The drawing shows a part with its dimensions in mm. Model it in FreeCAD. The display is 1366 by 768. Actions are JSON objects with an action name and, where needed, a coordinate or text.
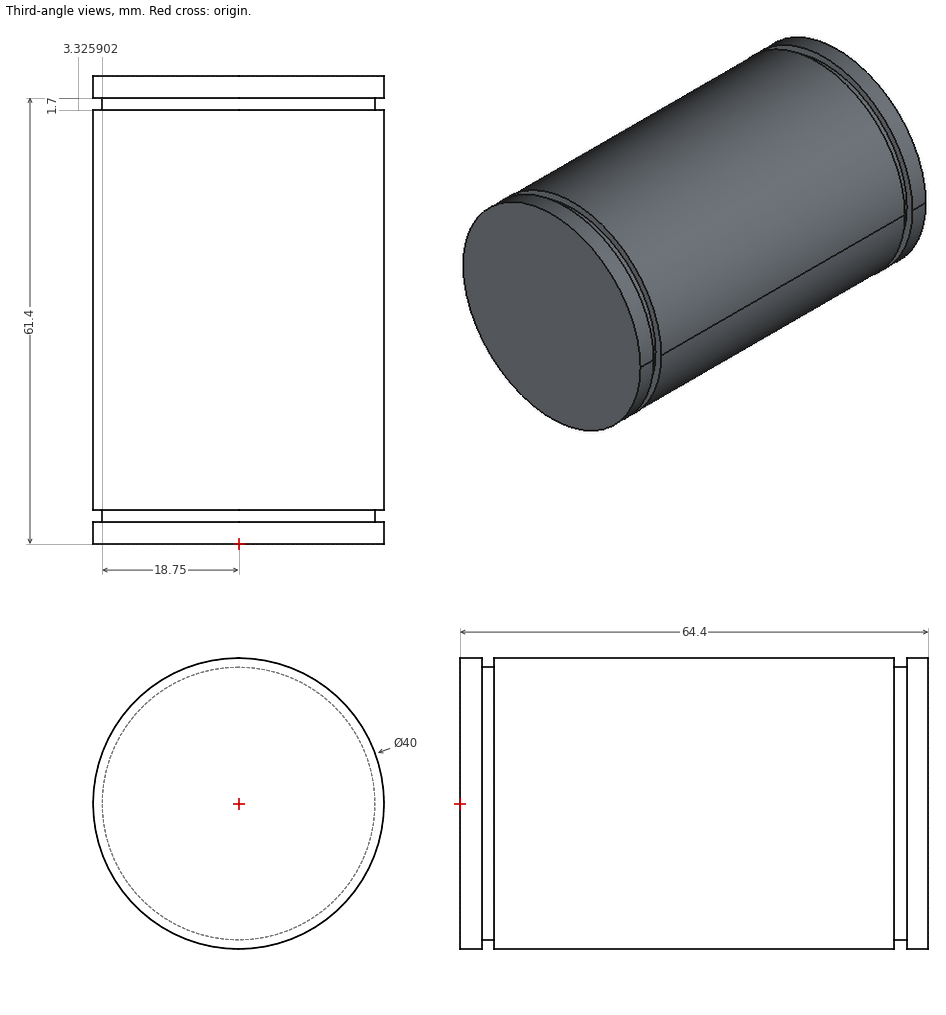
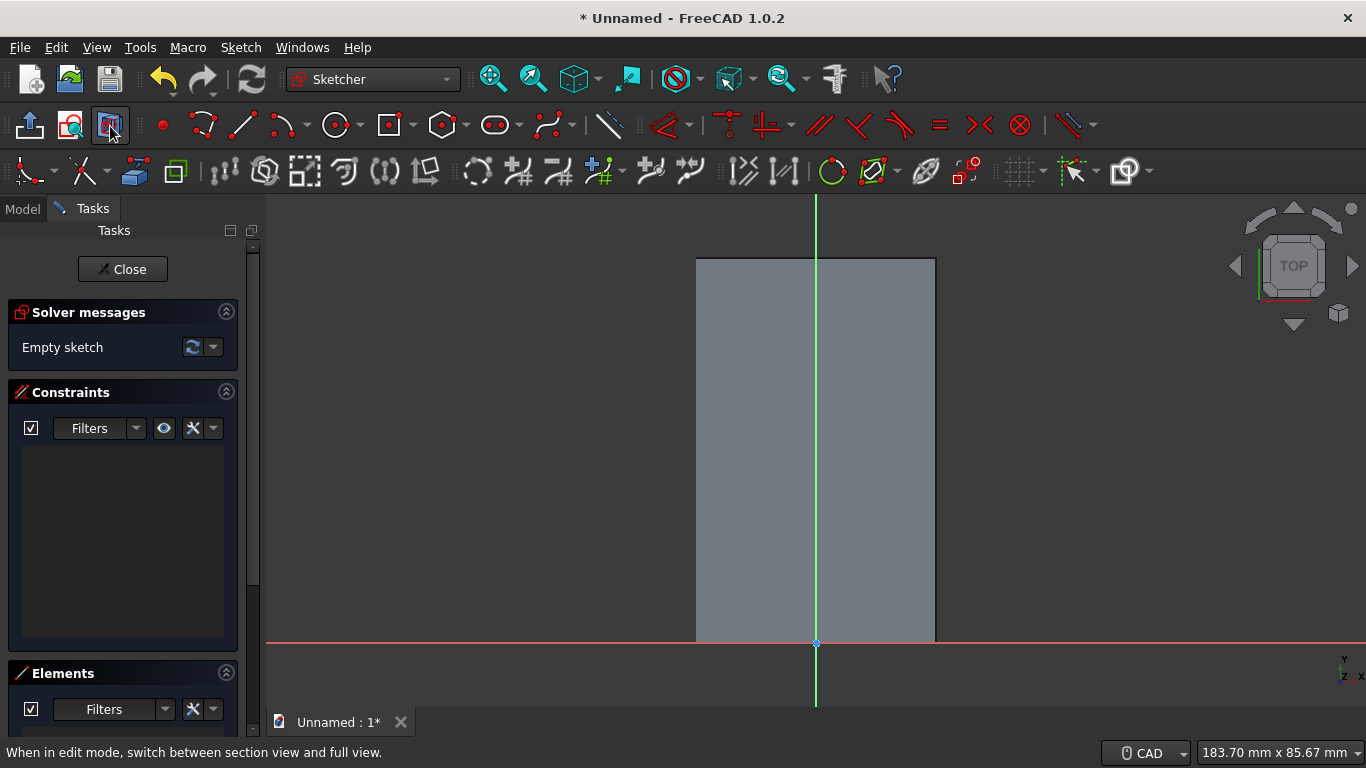
{"action": "scroll", "coordinate": [691, 272], "scroll_direction": "up", "scroll_amount": 15}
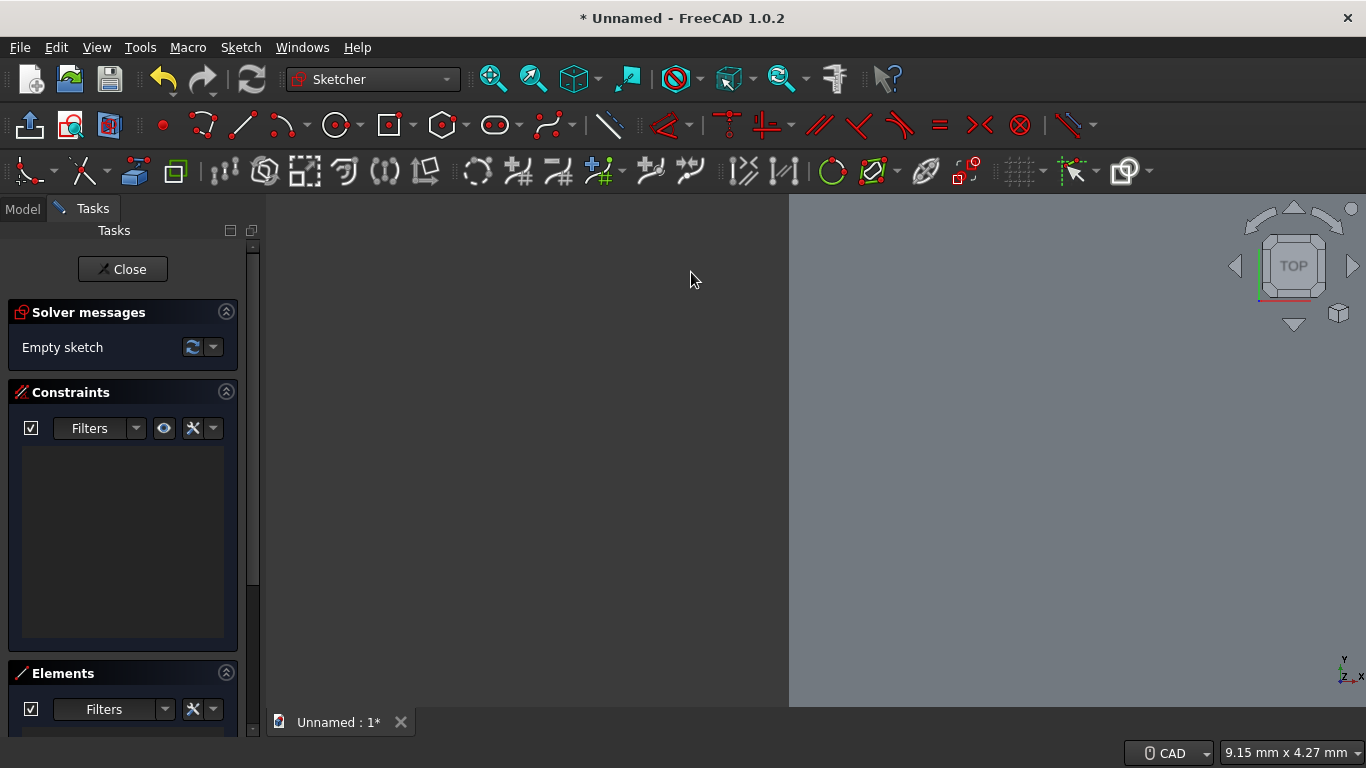
{"action": "scroll", "coordinate": [722, 433], "scroll_direction": "up", "scroll_amount": 2}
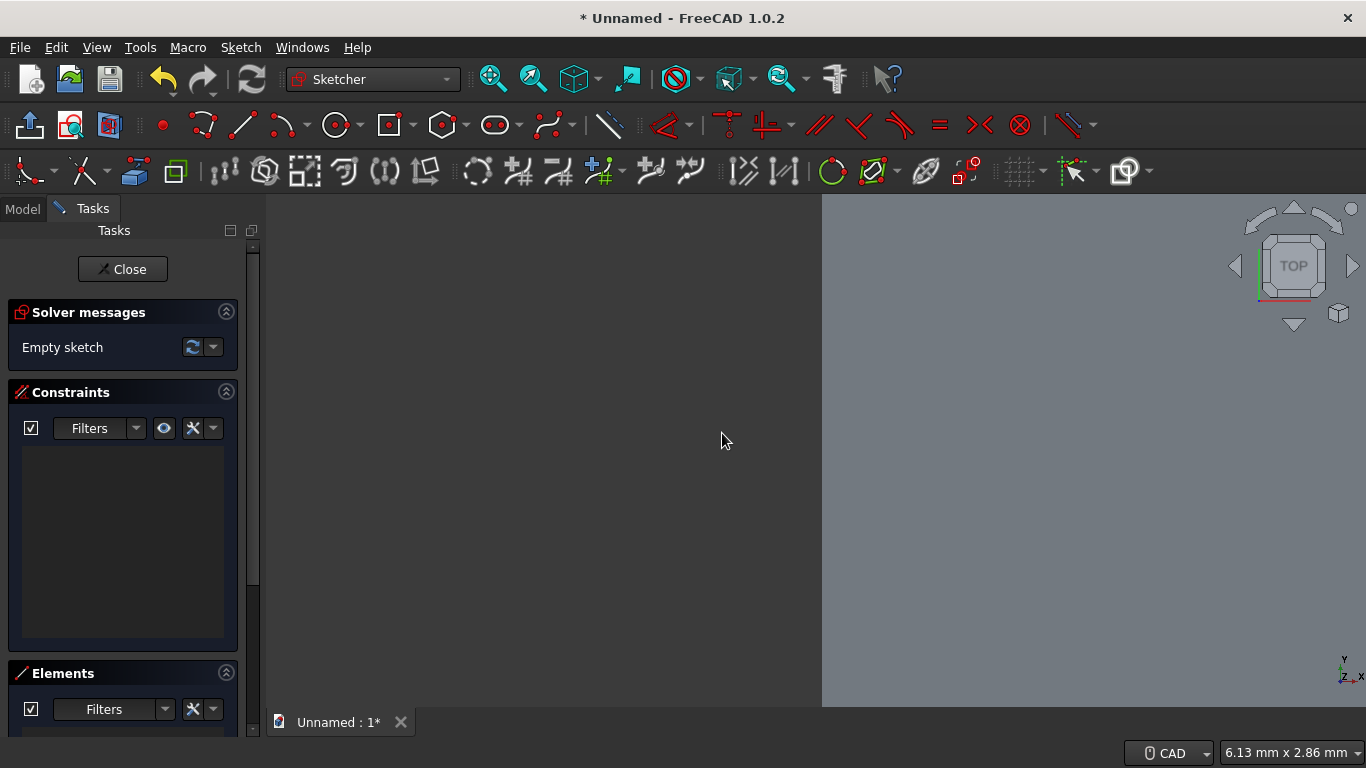
{"action": "key", "text": "g r"}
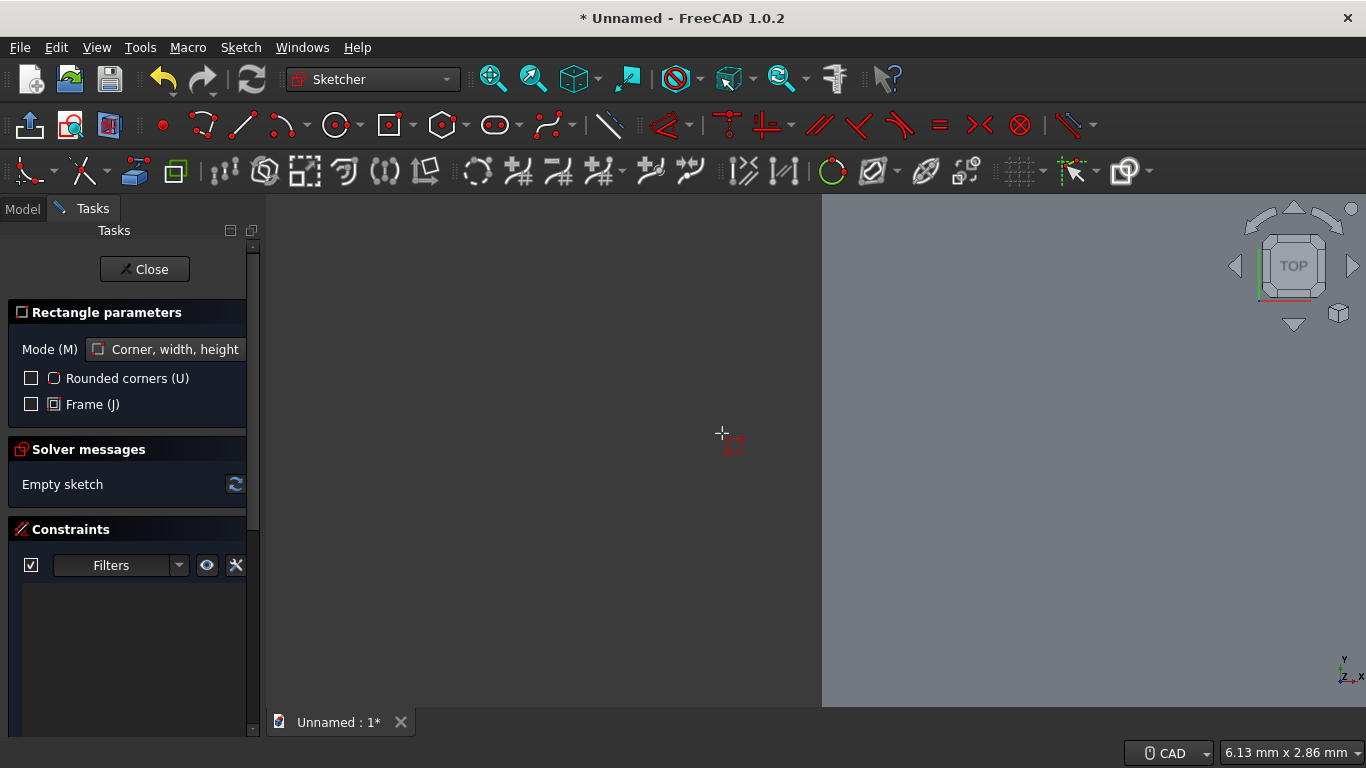
{"action": "left_click", "coordinate": [449, 298]}
{"action": "mouse_move", "coordinate": [1046, 603]}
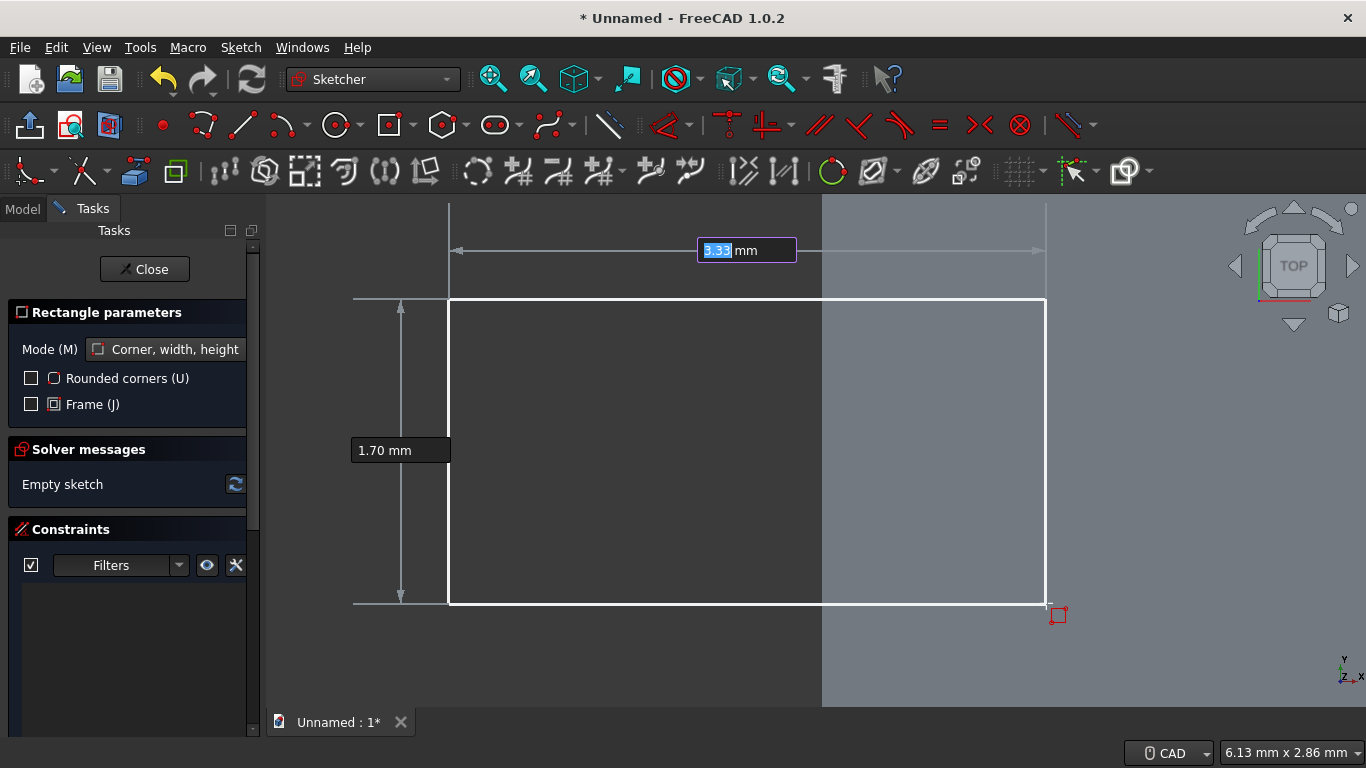
{"action": "type", "text": "3.325902"}
{"action": "key", "text": "Tab"}
{"action": "type", "text": "1.7"}
{"action": "key", "text": "Return"}
{"action": "key", "text": "Escape"}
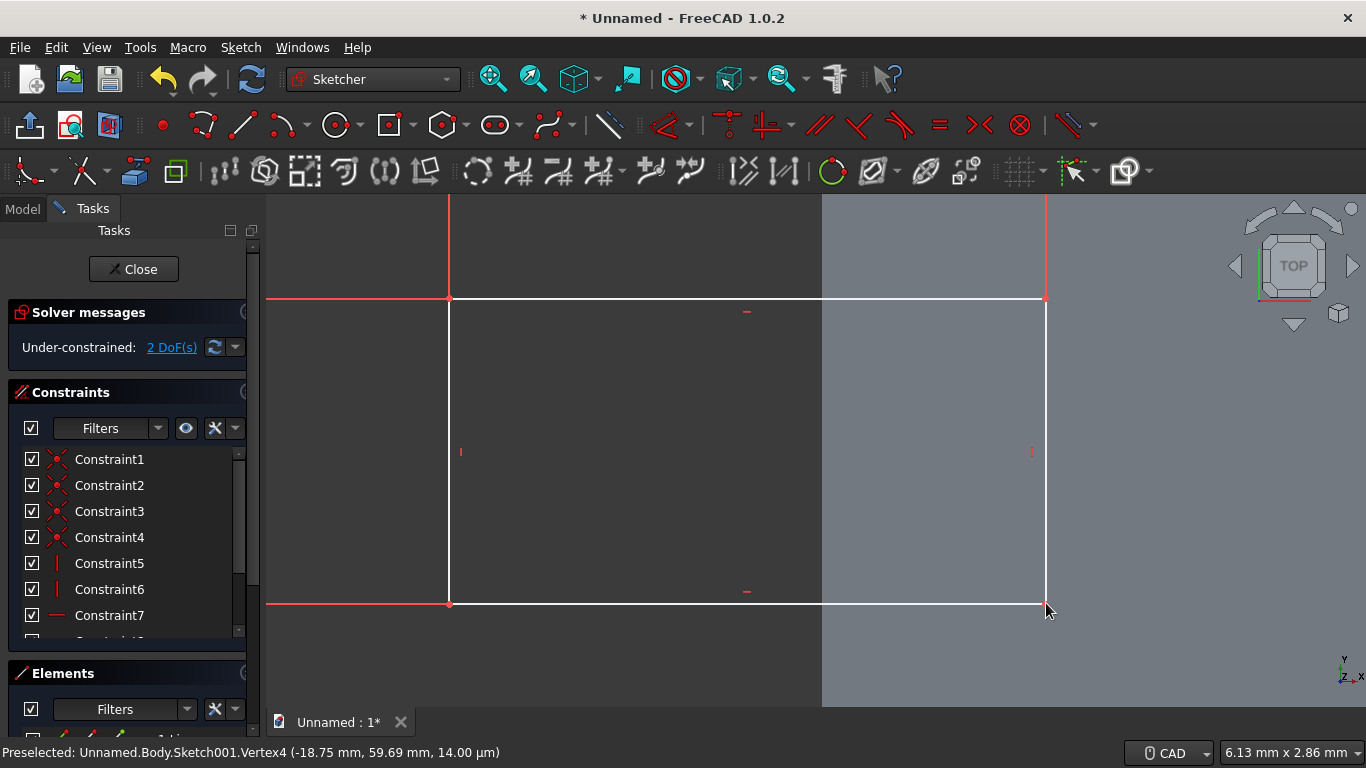
{"action": "left_click", "coordinate": [449, 299]}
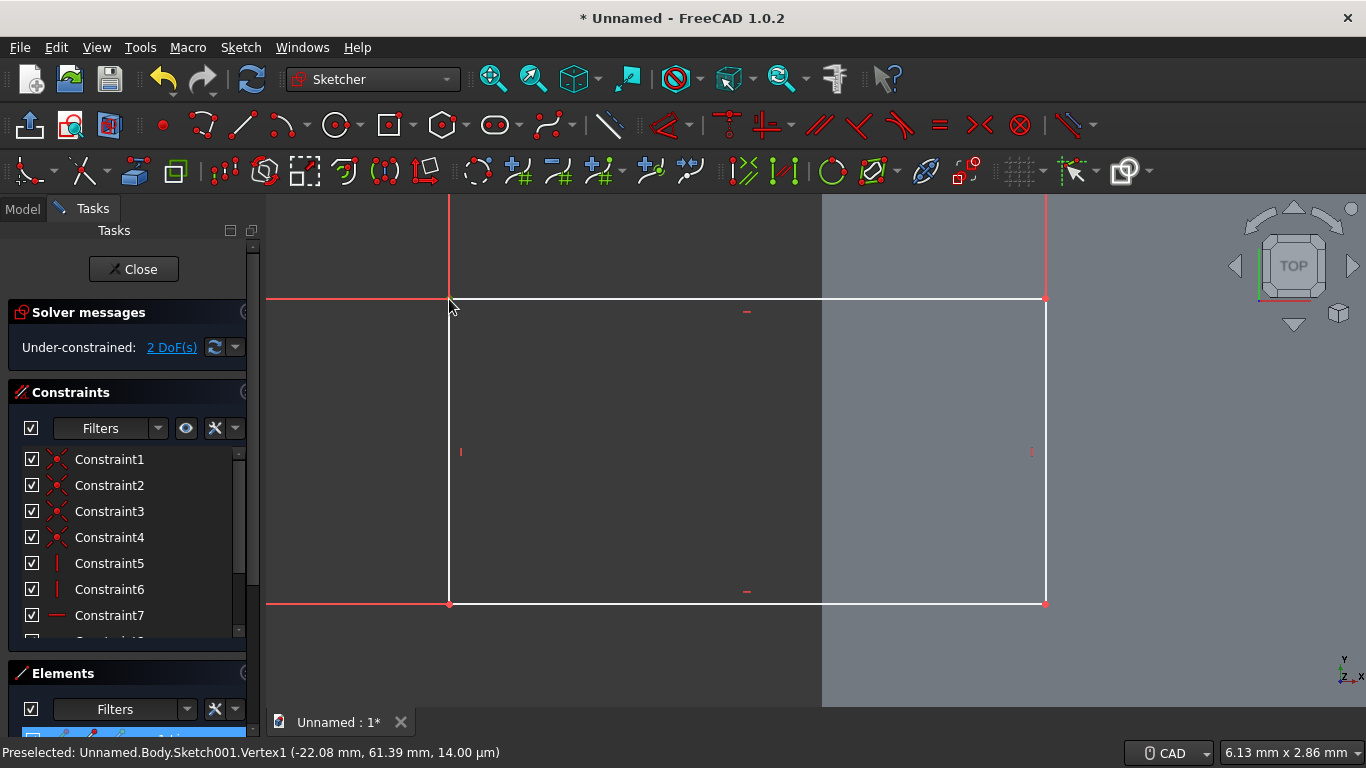
{"action": "key", "text": "i"}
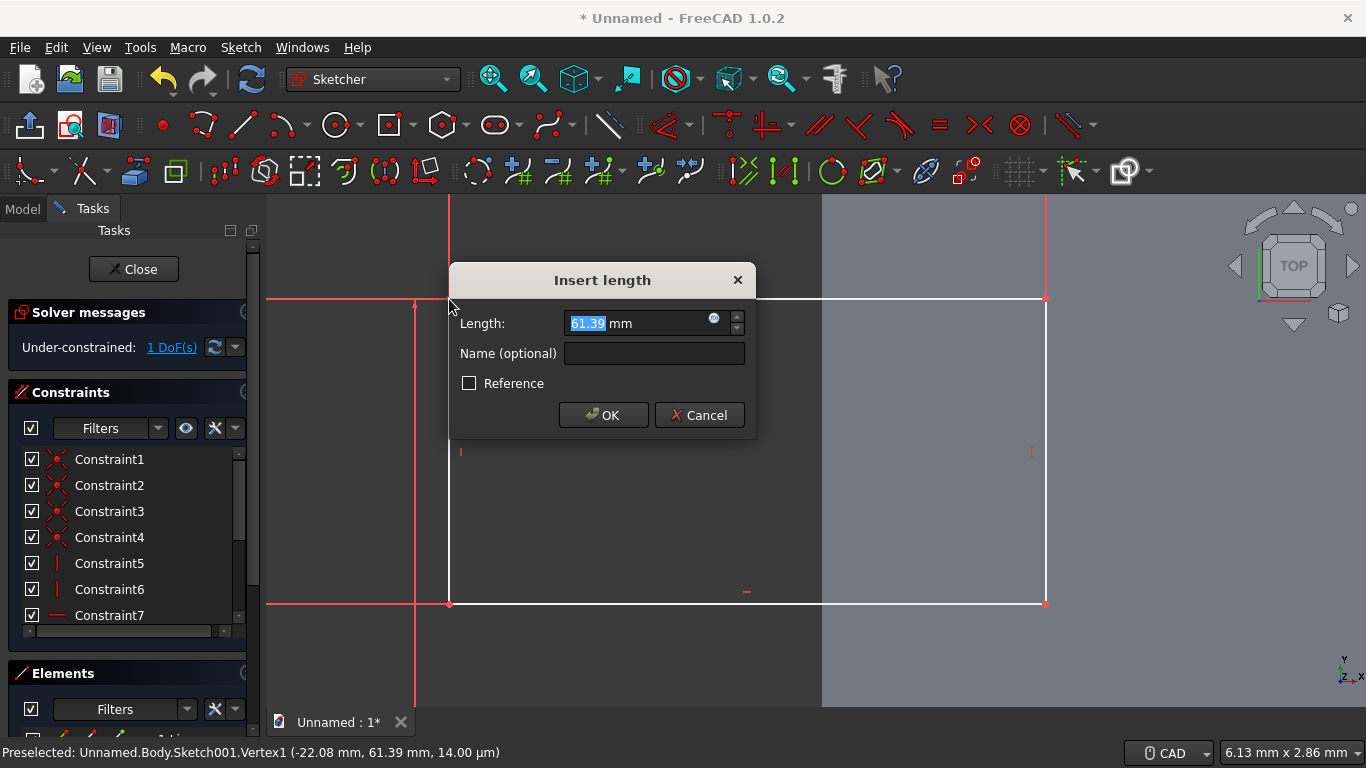
{"action": "type", "text": "61.4"}
{"action": "key", "text": "Return"}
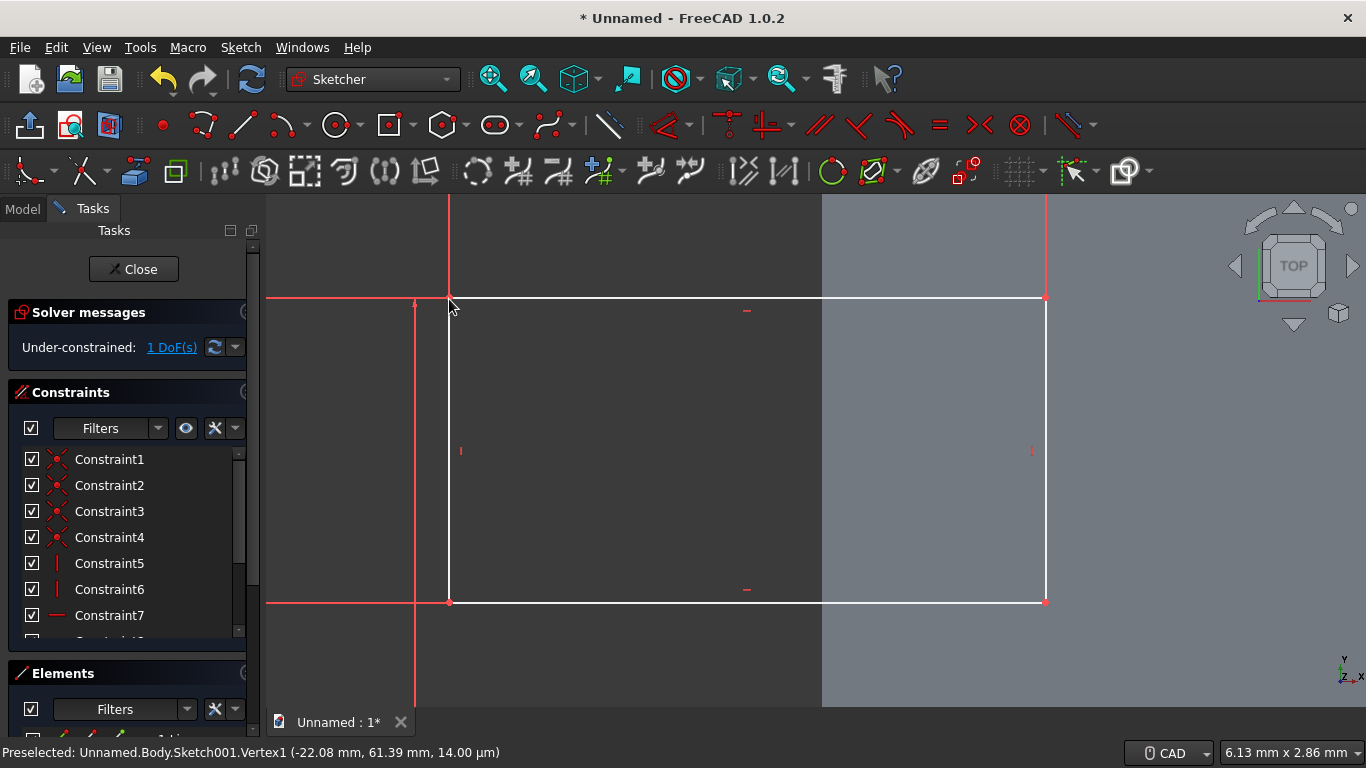
{"action": "left_click", "coordinate": [1046, 603]}